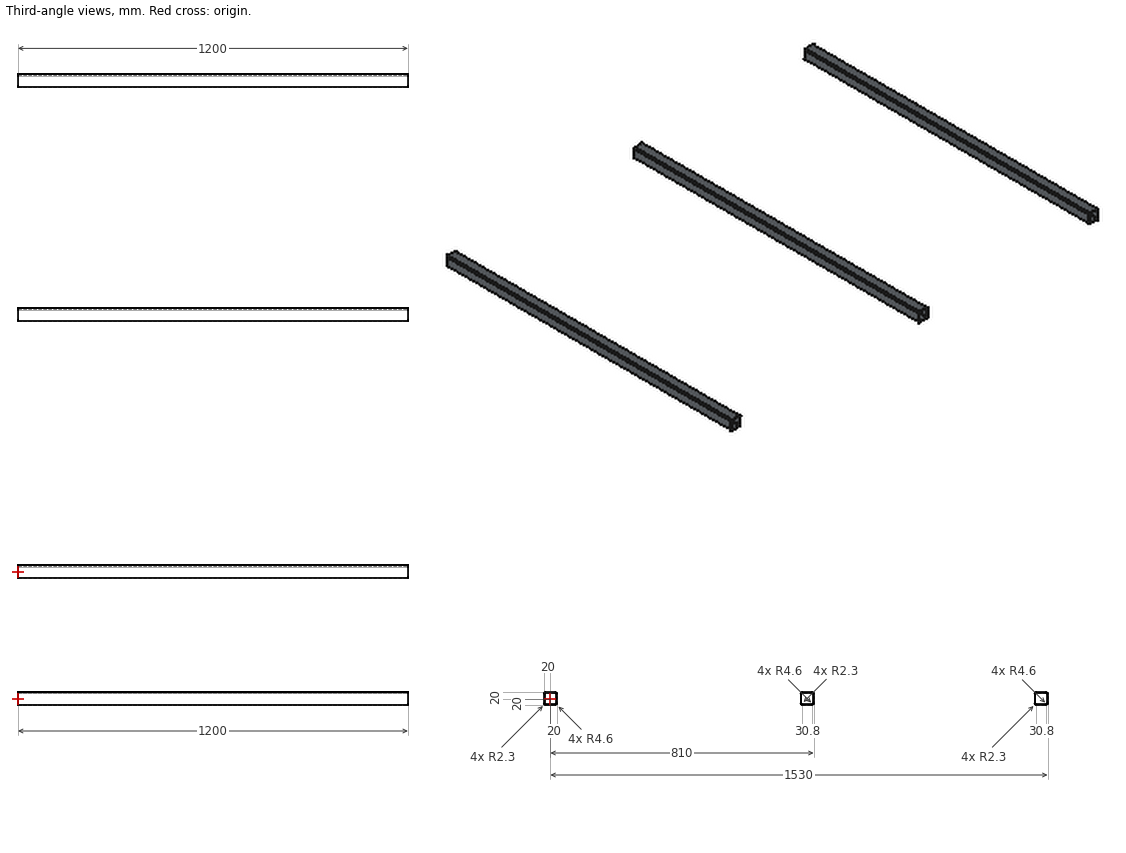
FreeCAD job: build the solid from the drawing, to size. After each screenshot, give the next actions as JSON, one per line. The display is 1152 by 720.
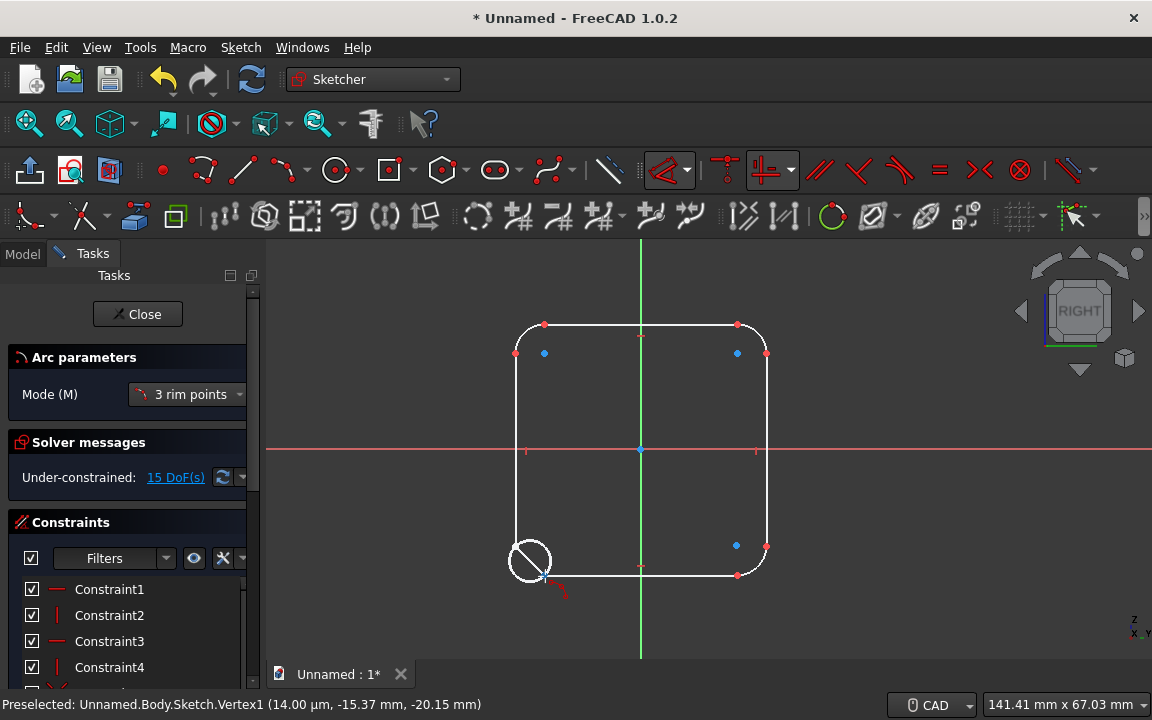
{"action": "scroll", "coordinate": [524, 566], "scroll_direction": "up", "scroll_amount": 4}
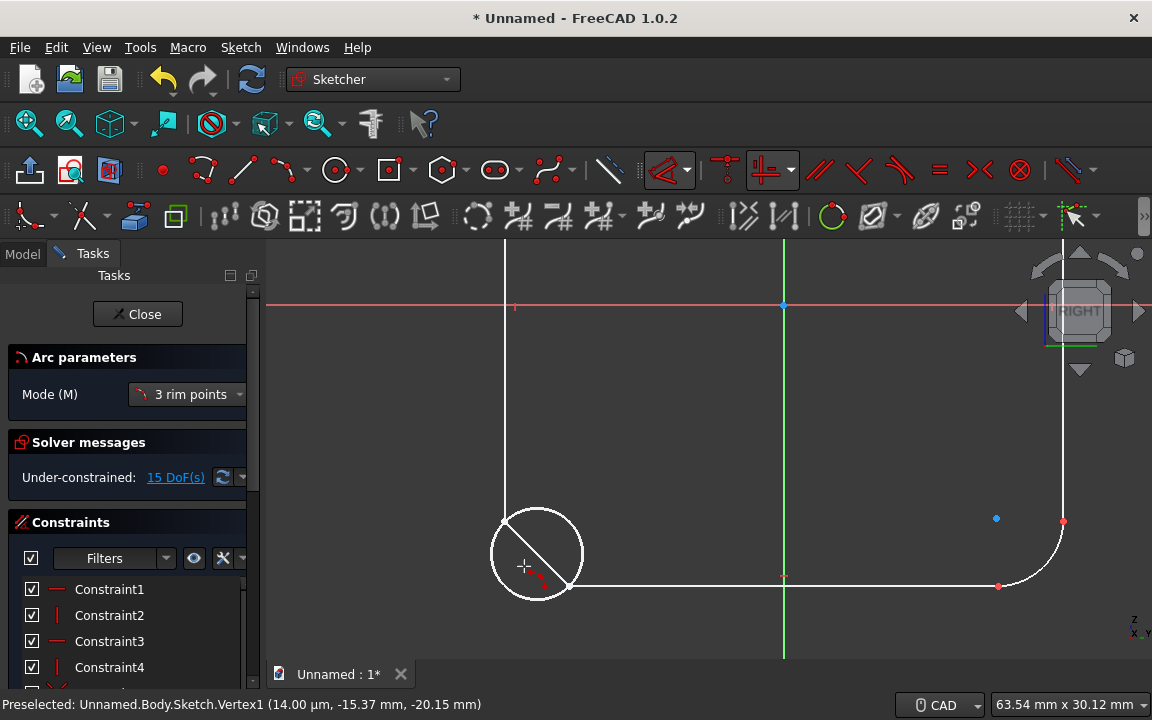
{"action": "left_click", "coordinate": [524, 565]}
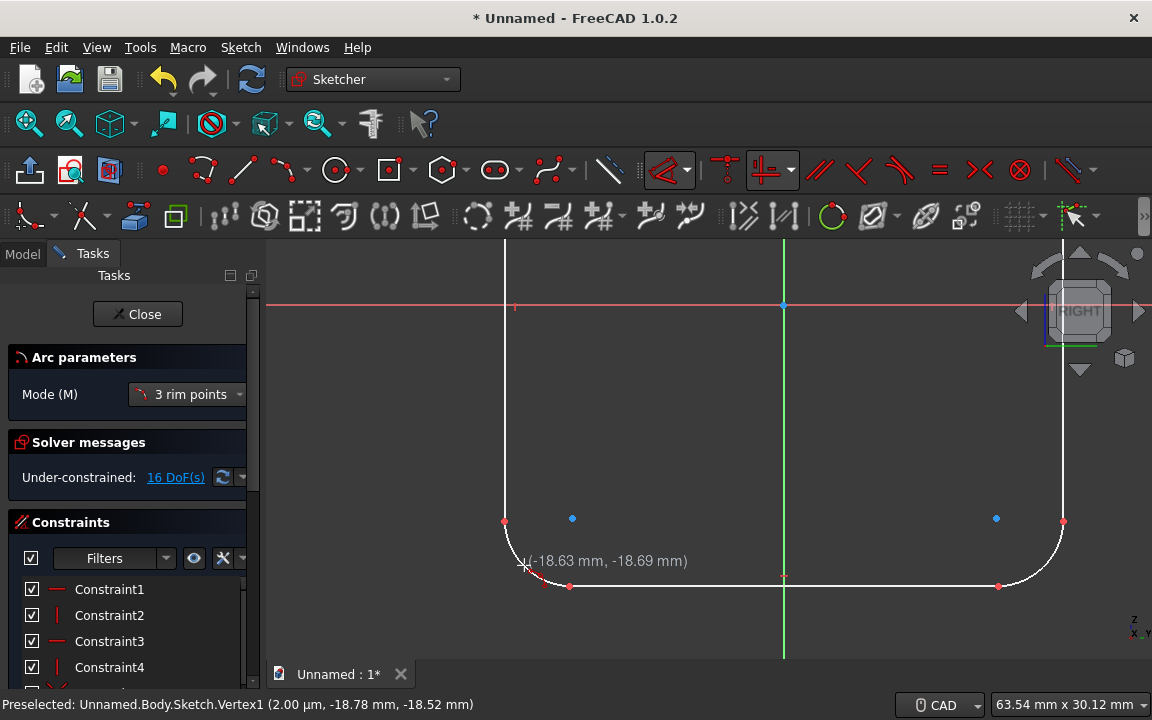
{"action": "key", "text": "g l"}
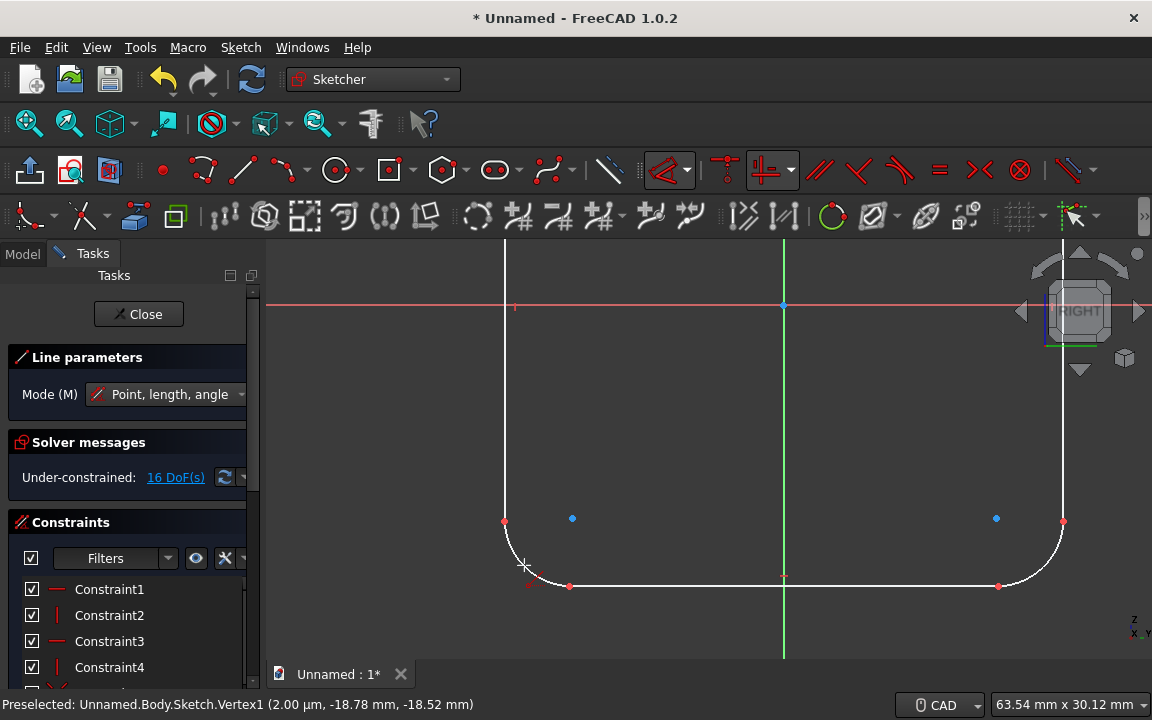
{"action": "scroll", "coordinate": [524, 566], "scroll_direction": "down", "scroll_amount": 4}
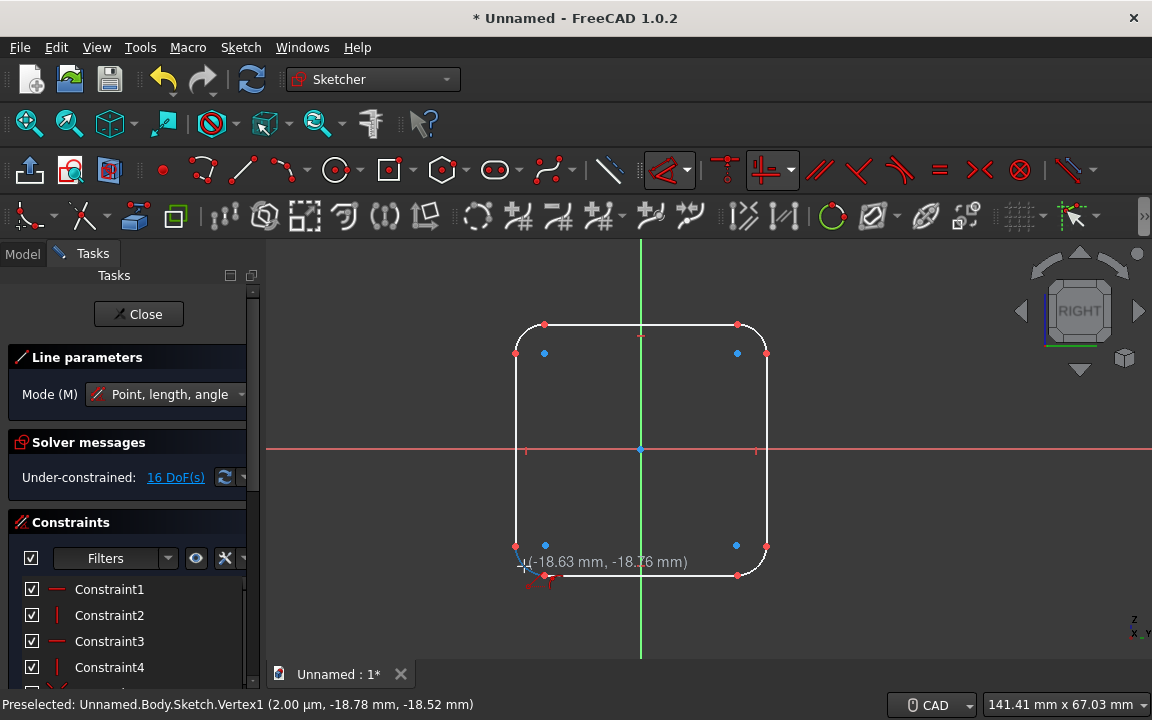
{"action": "left_click", "coordinate": [737, 560]}
{"action": "left_click", "coordinate": [544, 560]}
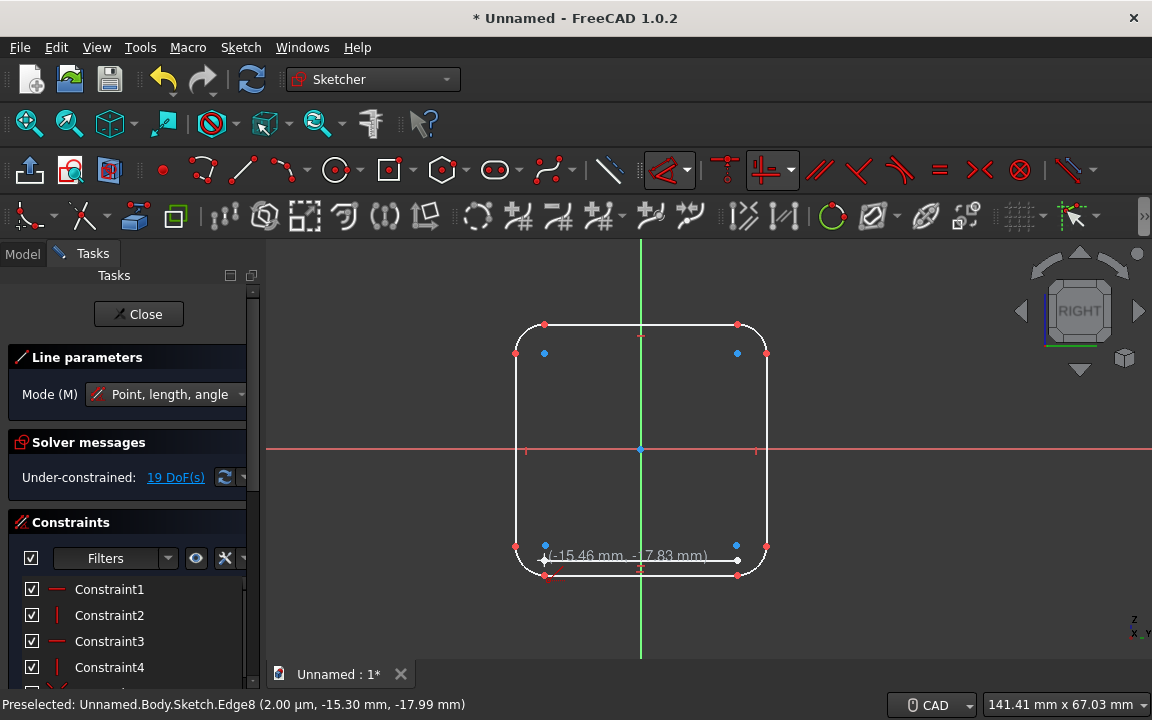
{"action": "left_click", "coordinate": [530, 546]}
{"action": "left_click", "coordinate": [530, 353]}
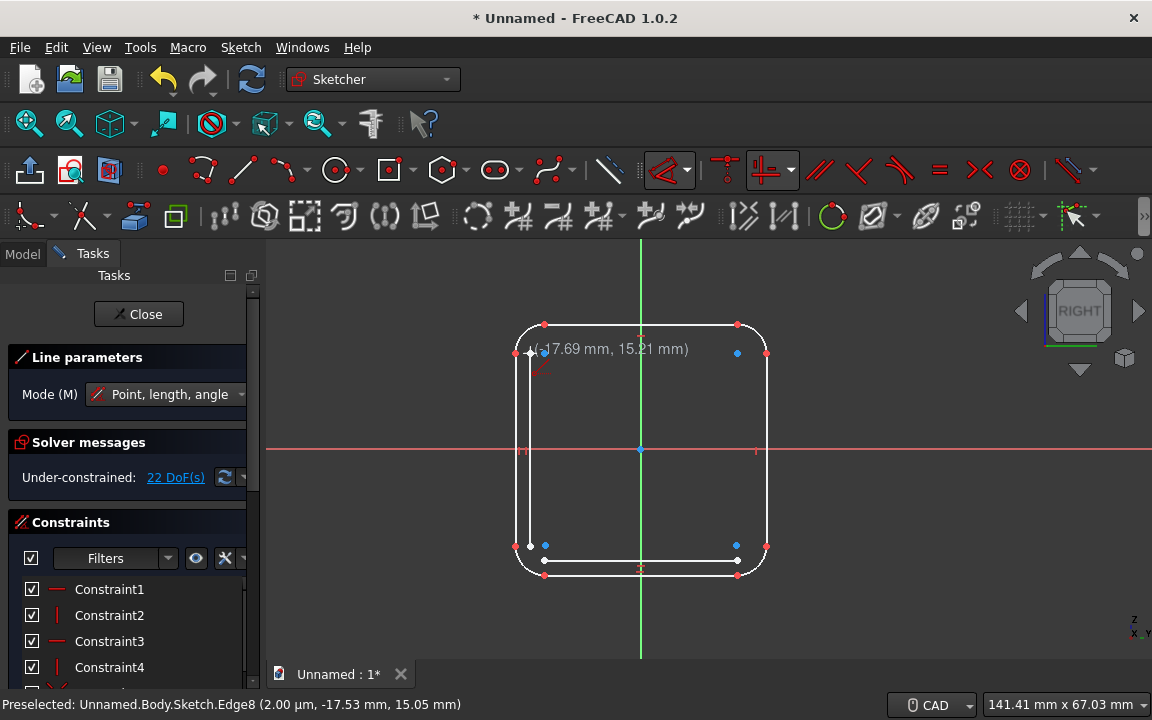
{"action": "left_click", "coordinate": [544, 338]}
{"action": "left_click", "coordinate": [737, 338]}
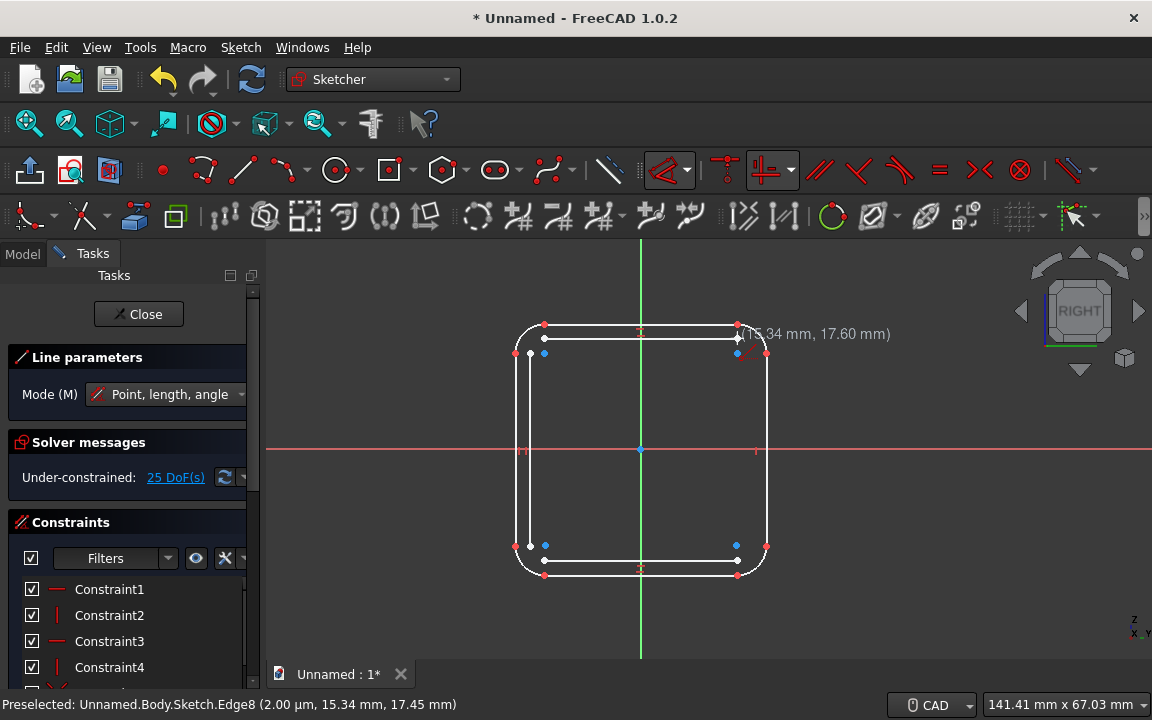
{"action": "left_click", "coordinate": [752, 353]}
{"action": "left_click", "coordinate": [752, 546]}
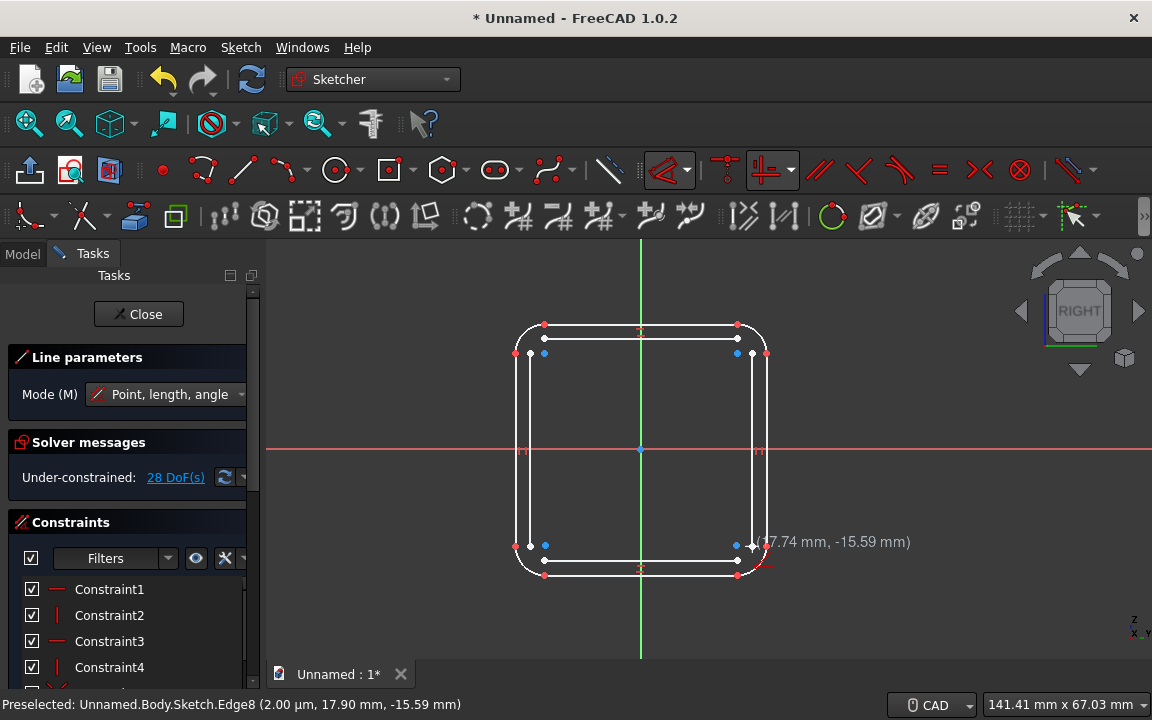
{"action": "key", "text": "g 3 a"}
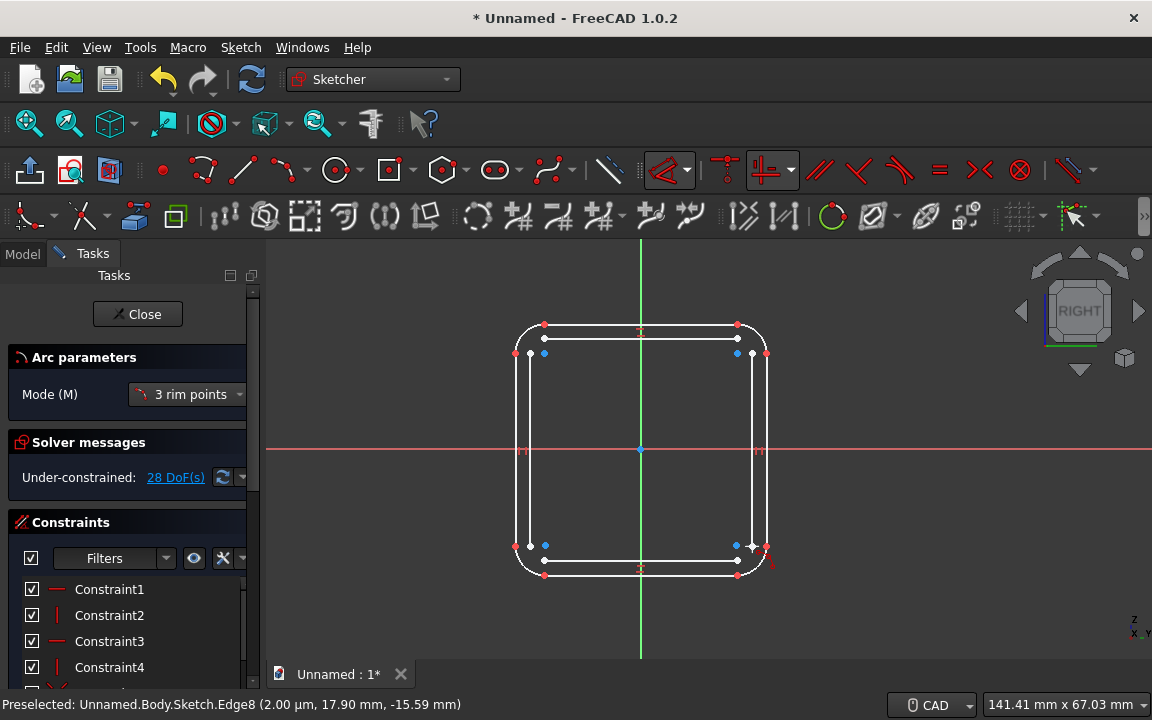
{"action": "left_click", "coordinate": [544, 561]}
{"action": "left_click", "coordinate": [530, 547]}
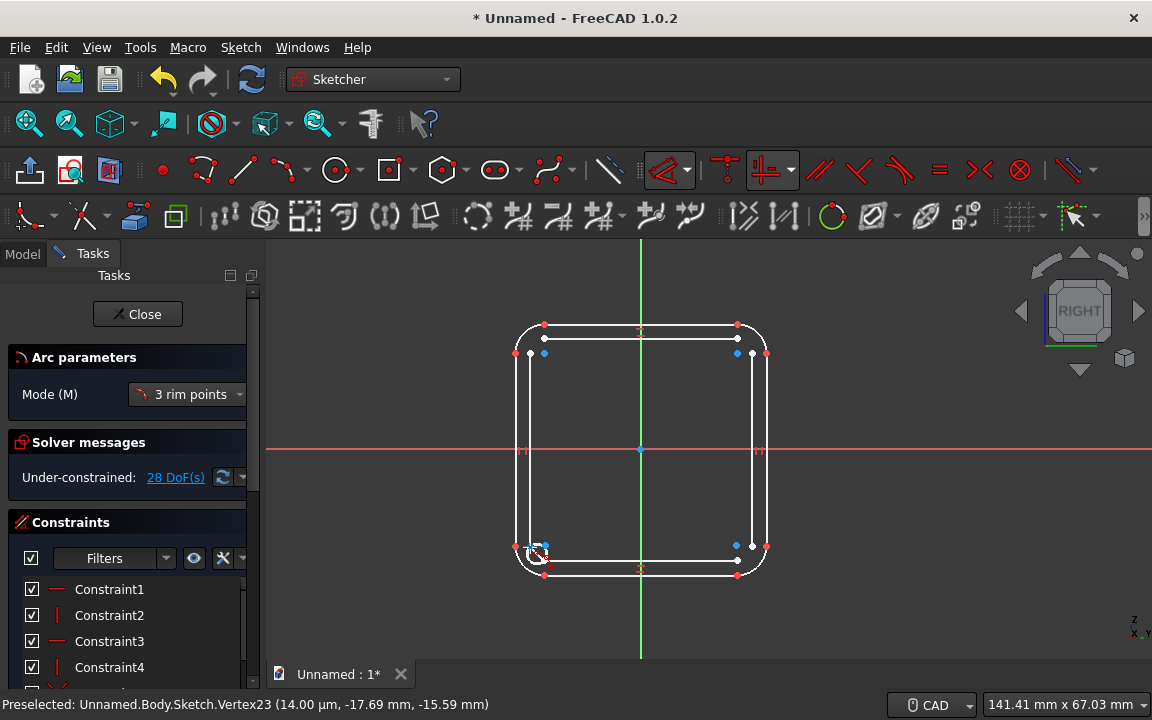
{"action": "scroll", "coordinate": [534, 556], "scroll_direction": "up", "scroll_amount": 7}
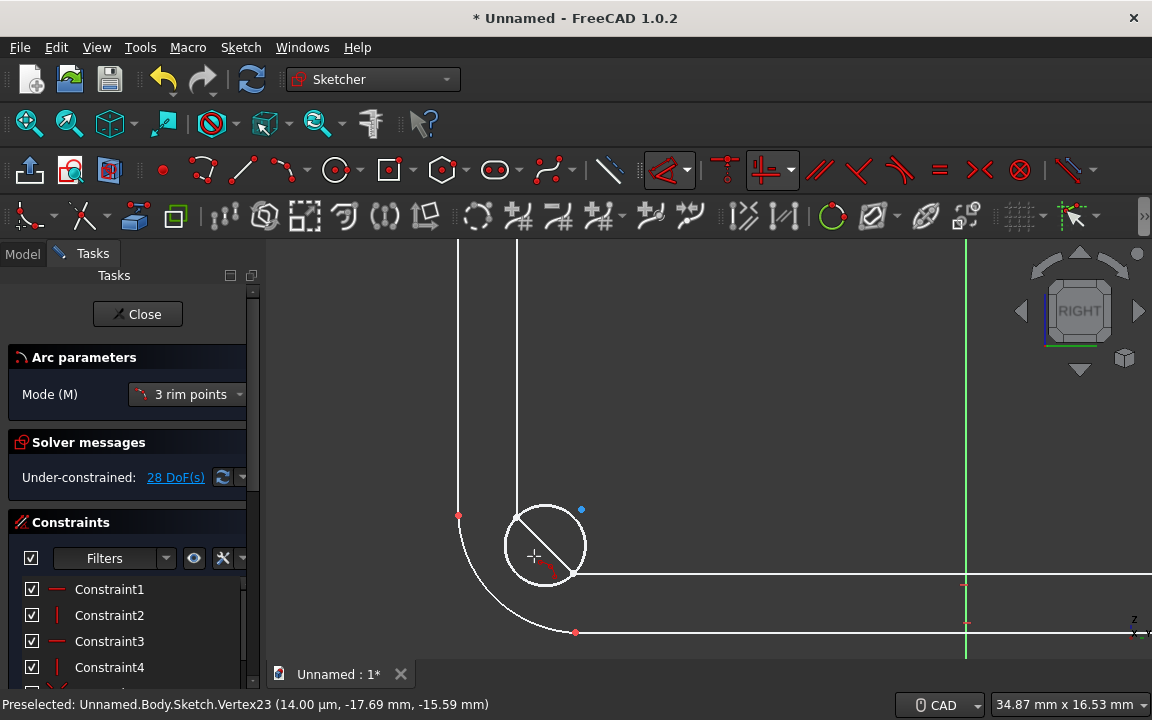
{"action": "left_click", "coordinate": [534, 554]}